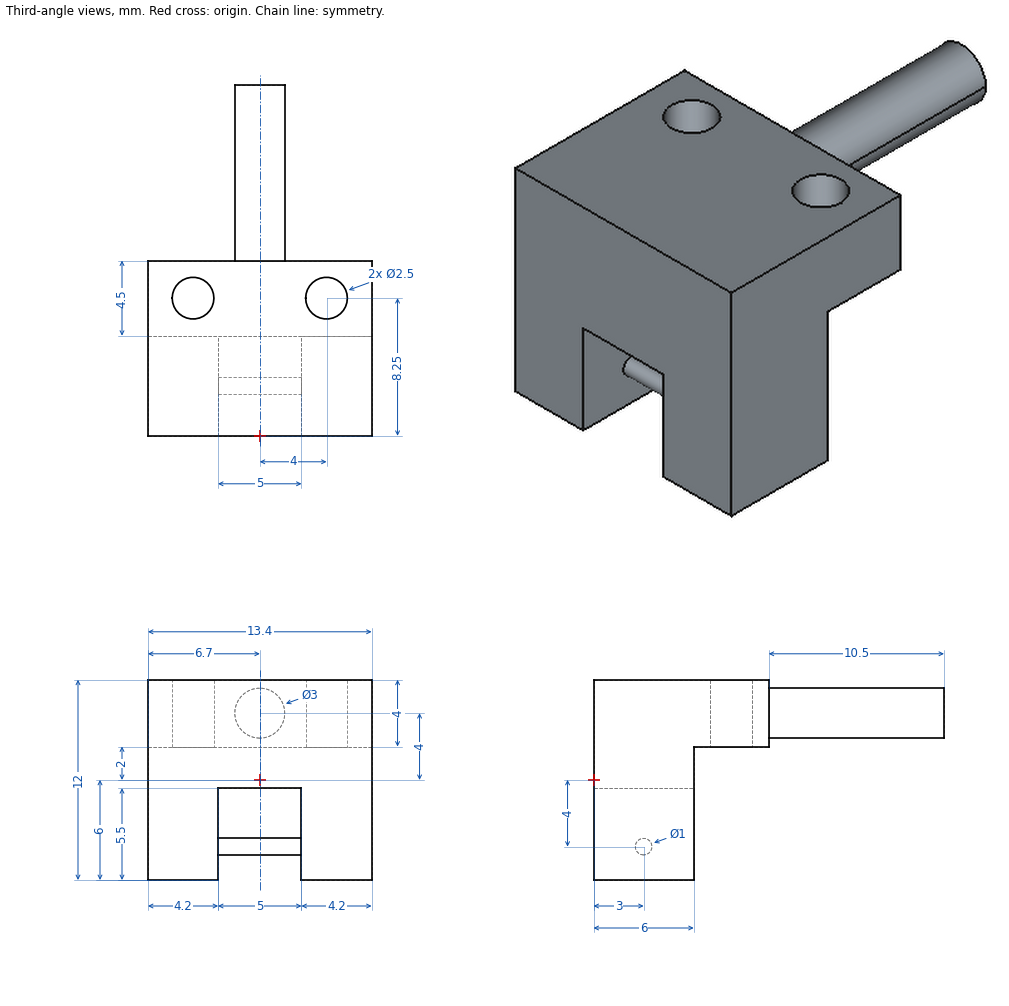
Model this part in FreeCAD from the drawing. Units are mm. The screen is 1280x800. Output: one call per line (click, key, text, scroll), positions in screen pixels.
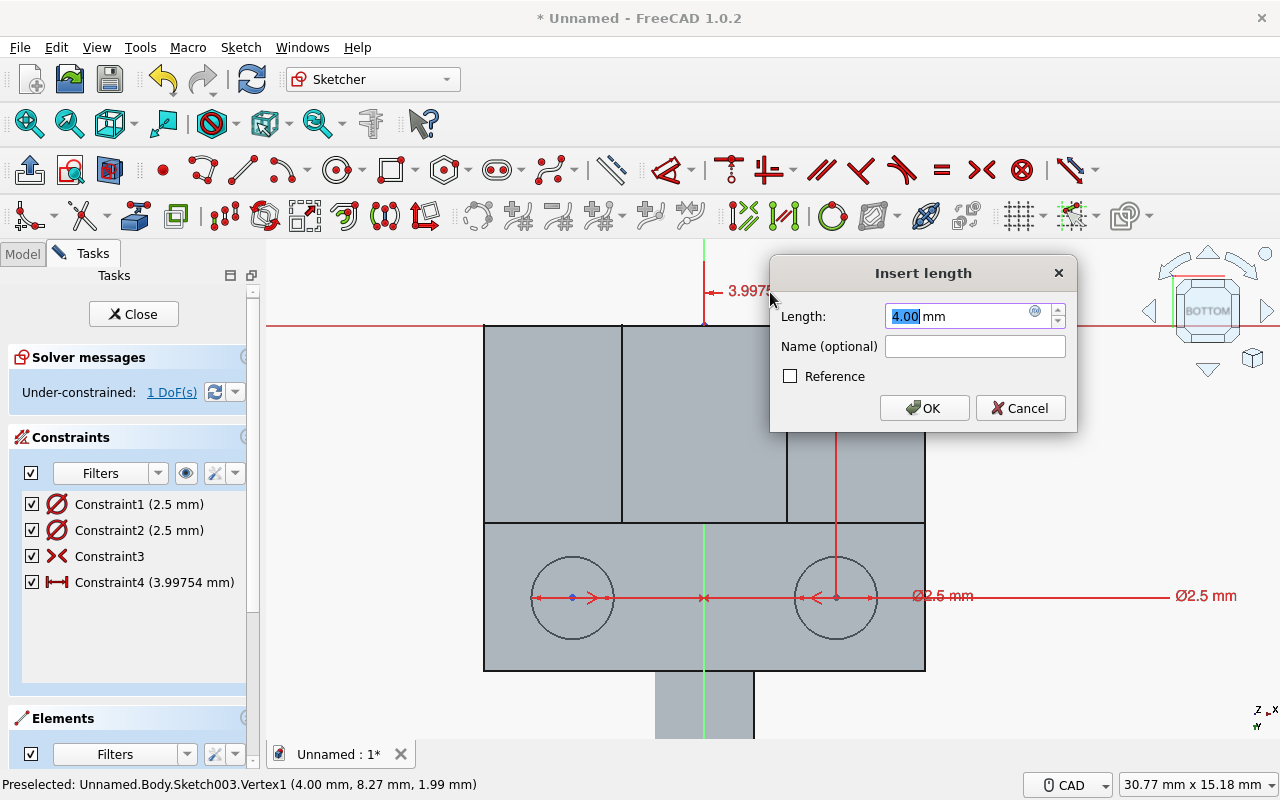
text(4)
key(Return)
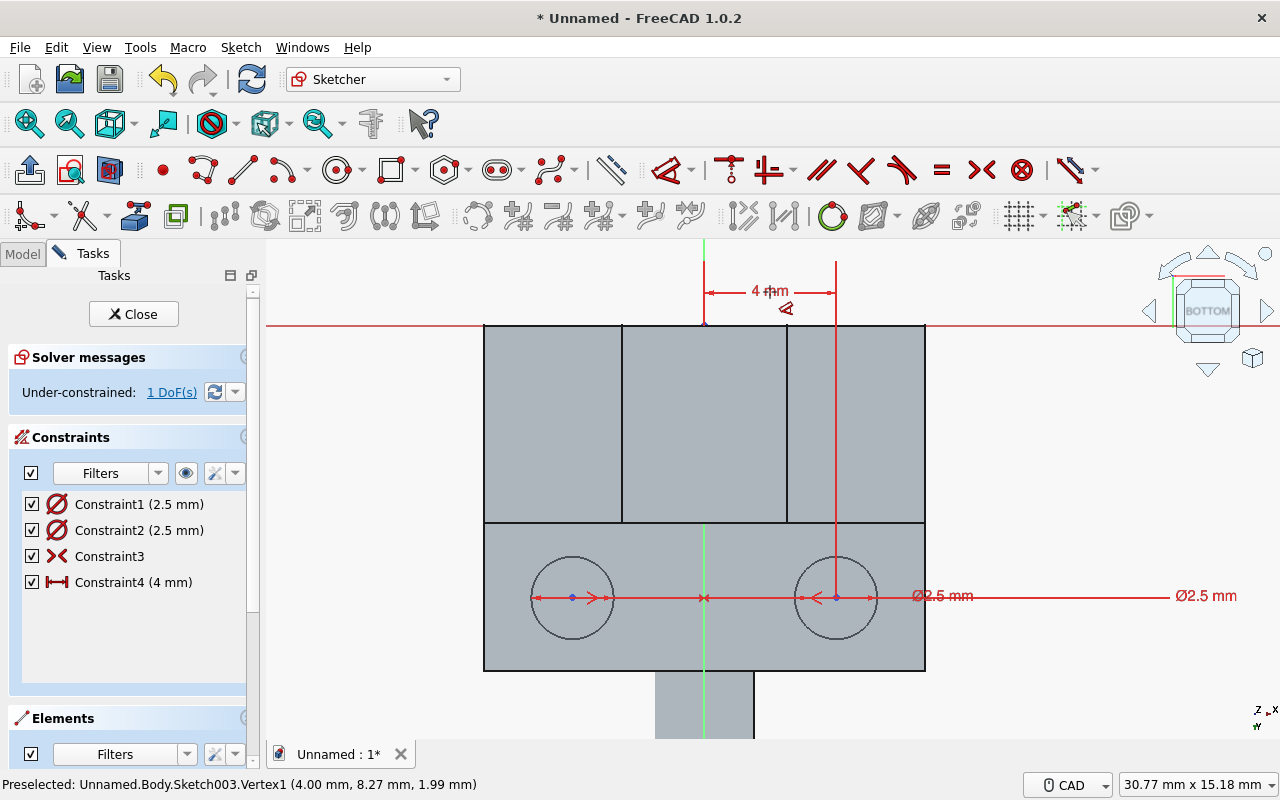
click(836, 598)
click(870, 462)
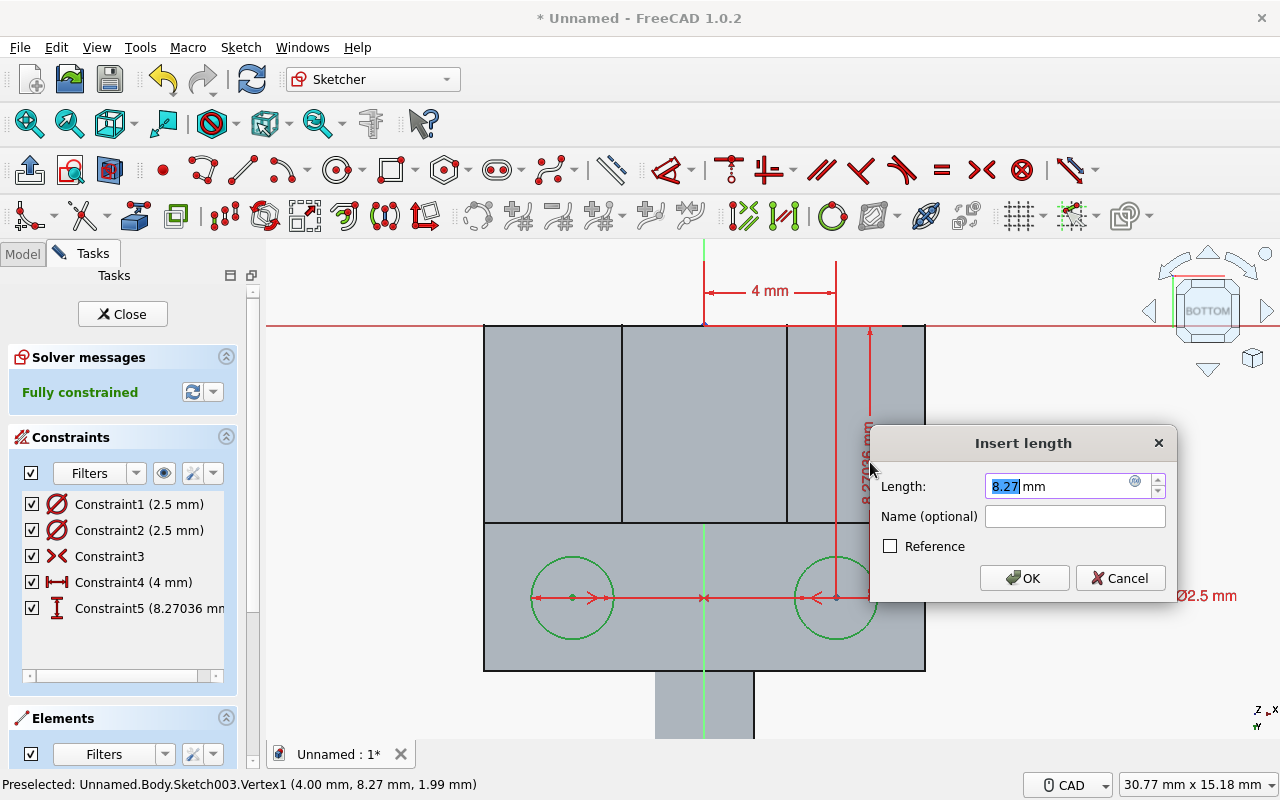
text(8.25)
key(Return)
key(Escape)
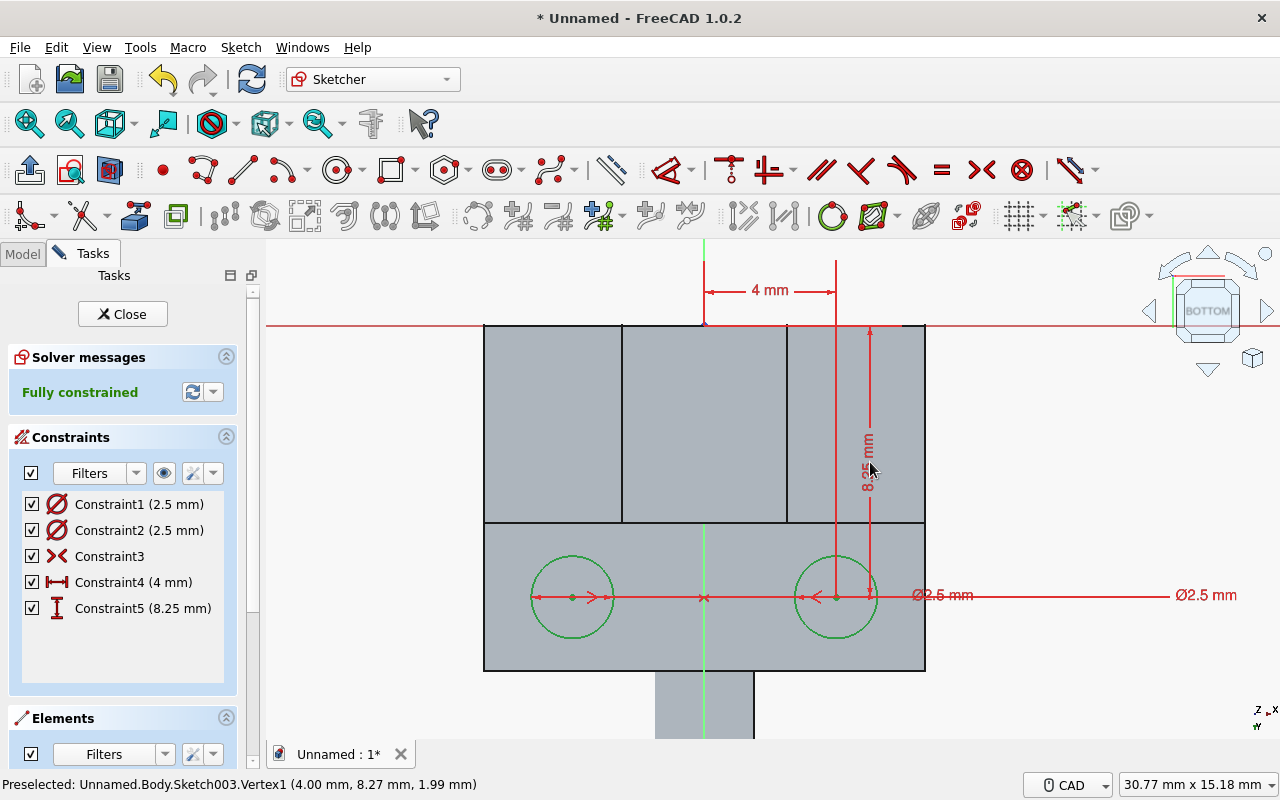
click(123, 314)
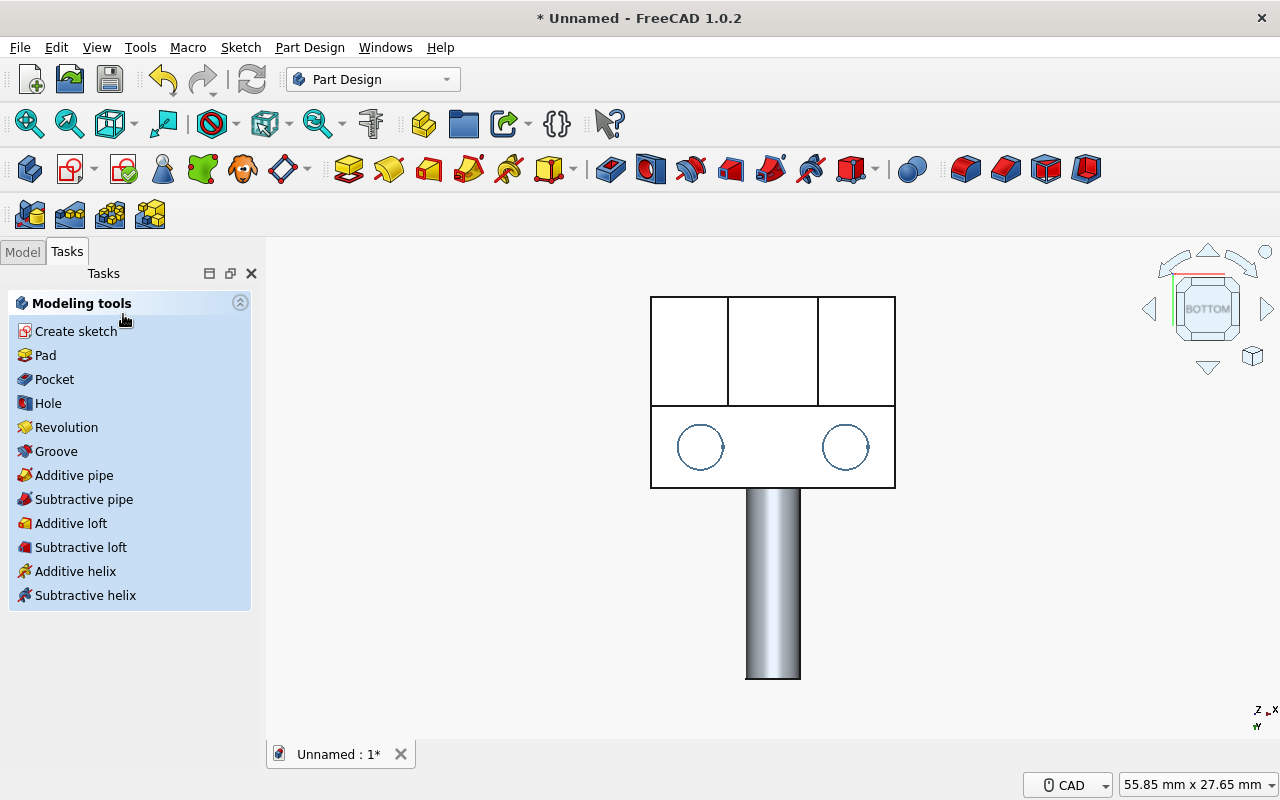
click(612, 170)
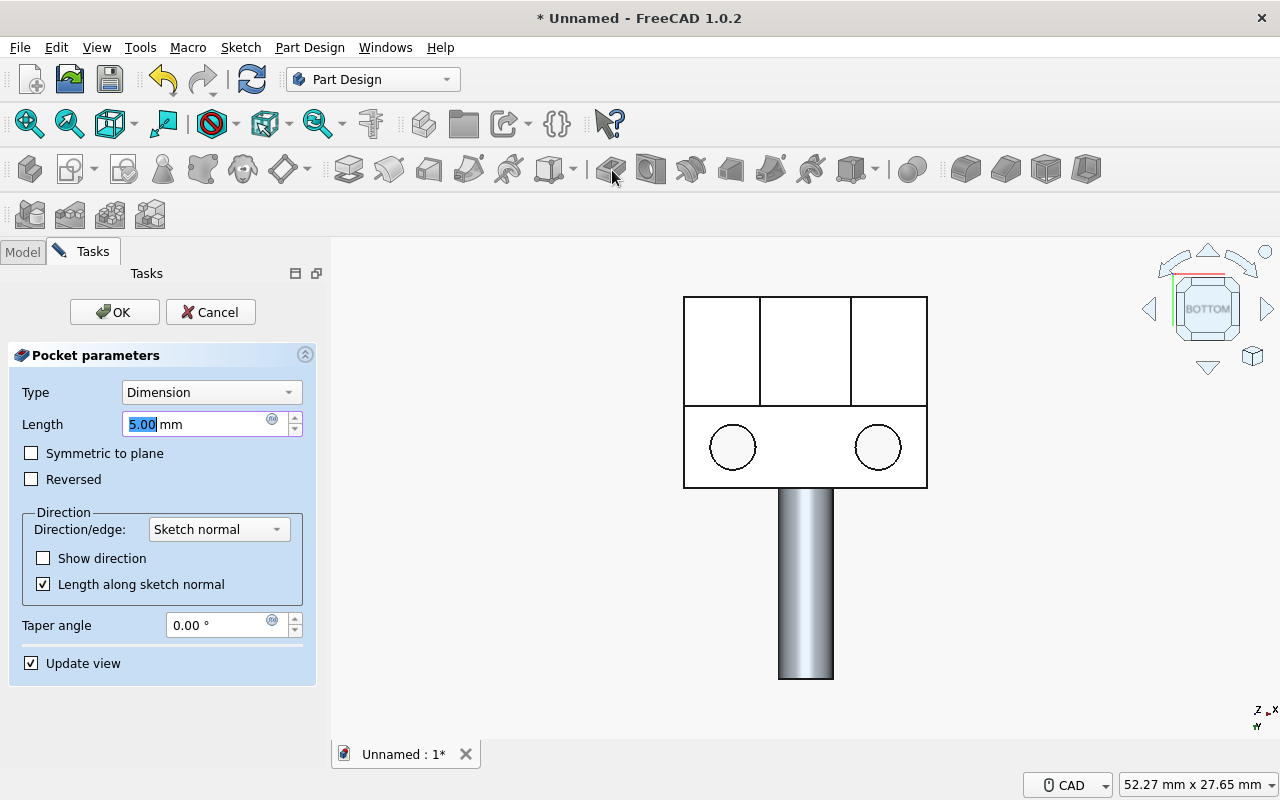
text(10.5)
key(Tab)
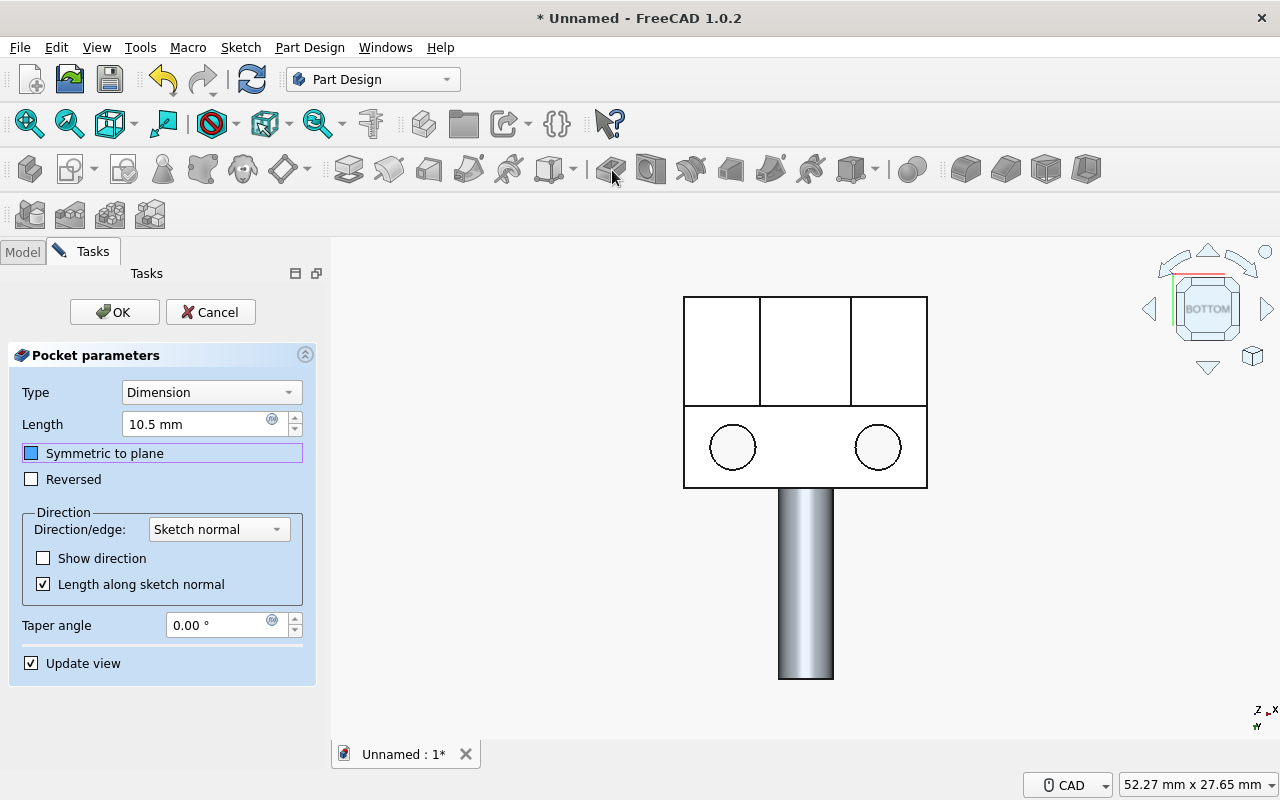
click(115, 312)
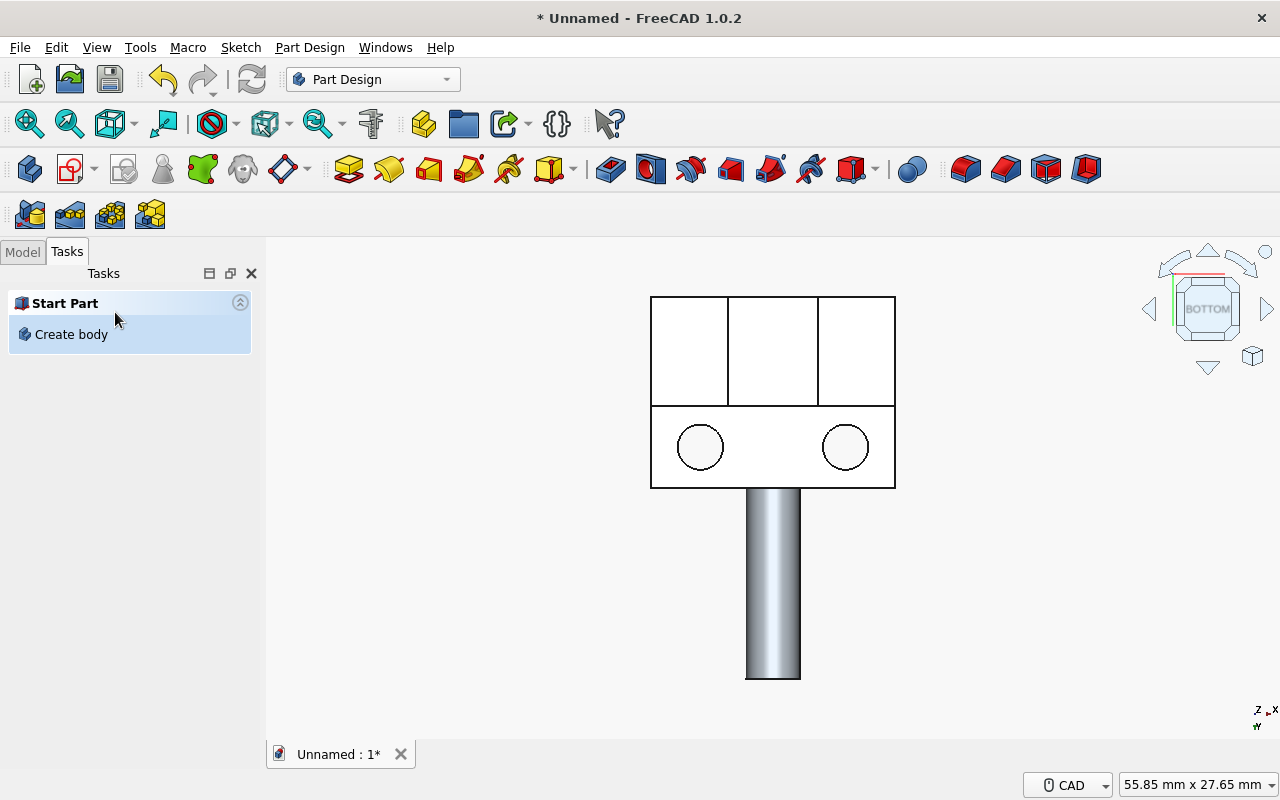
click(23, 251)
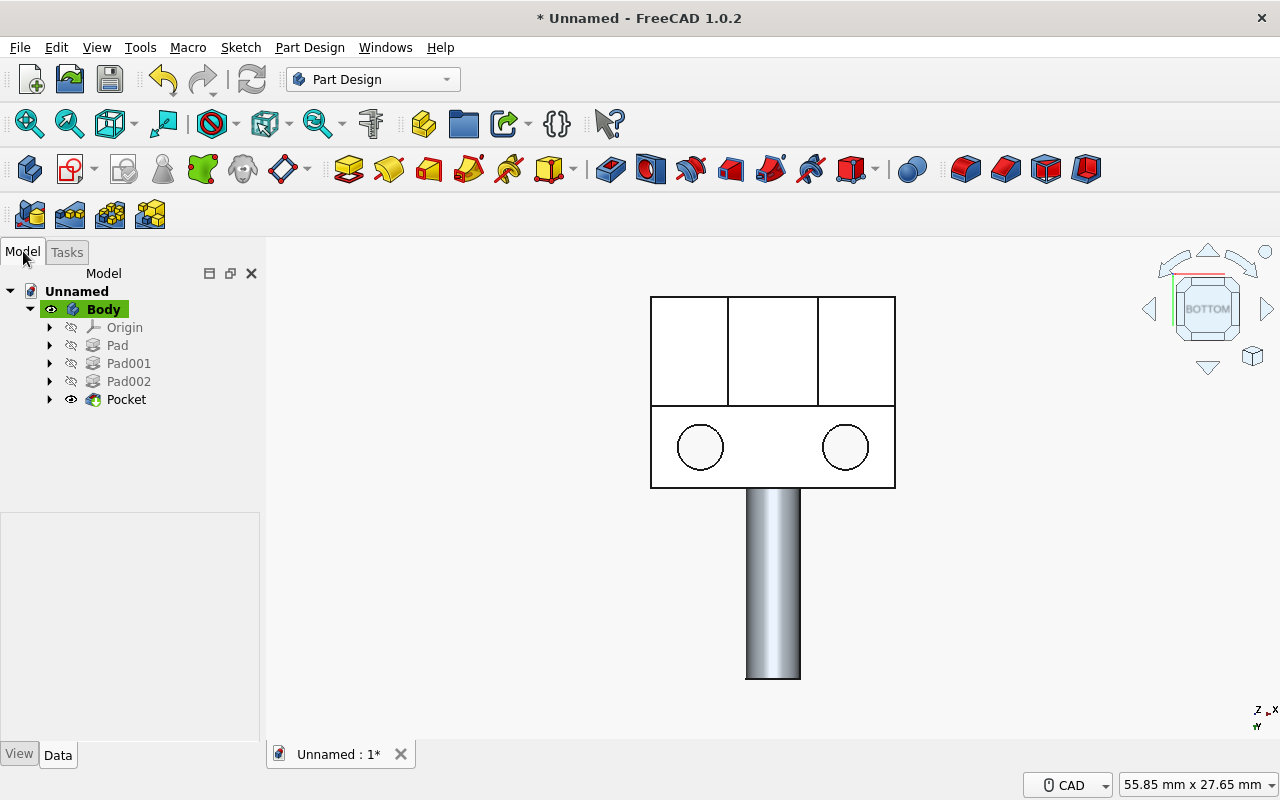
click(50, 327)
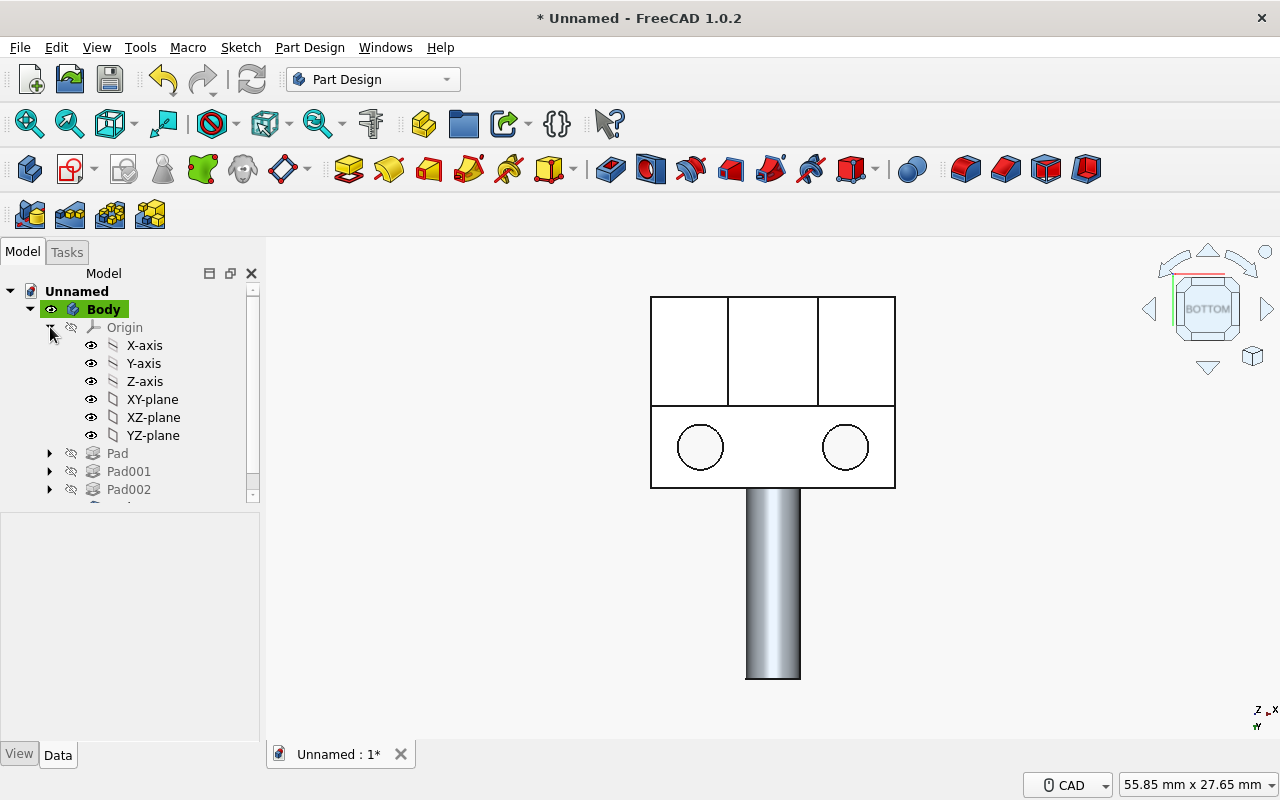
click(136, 435)